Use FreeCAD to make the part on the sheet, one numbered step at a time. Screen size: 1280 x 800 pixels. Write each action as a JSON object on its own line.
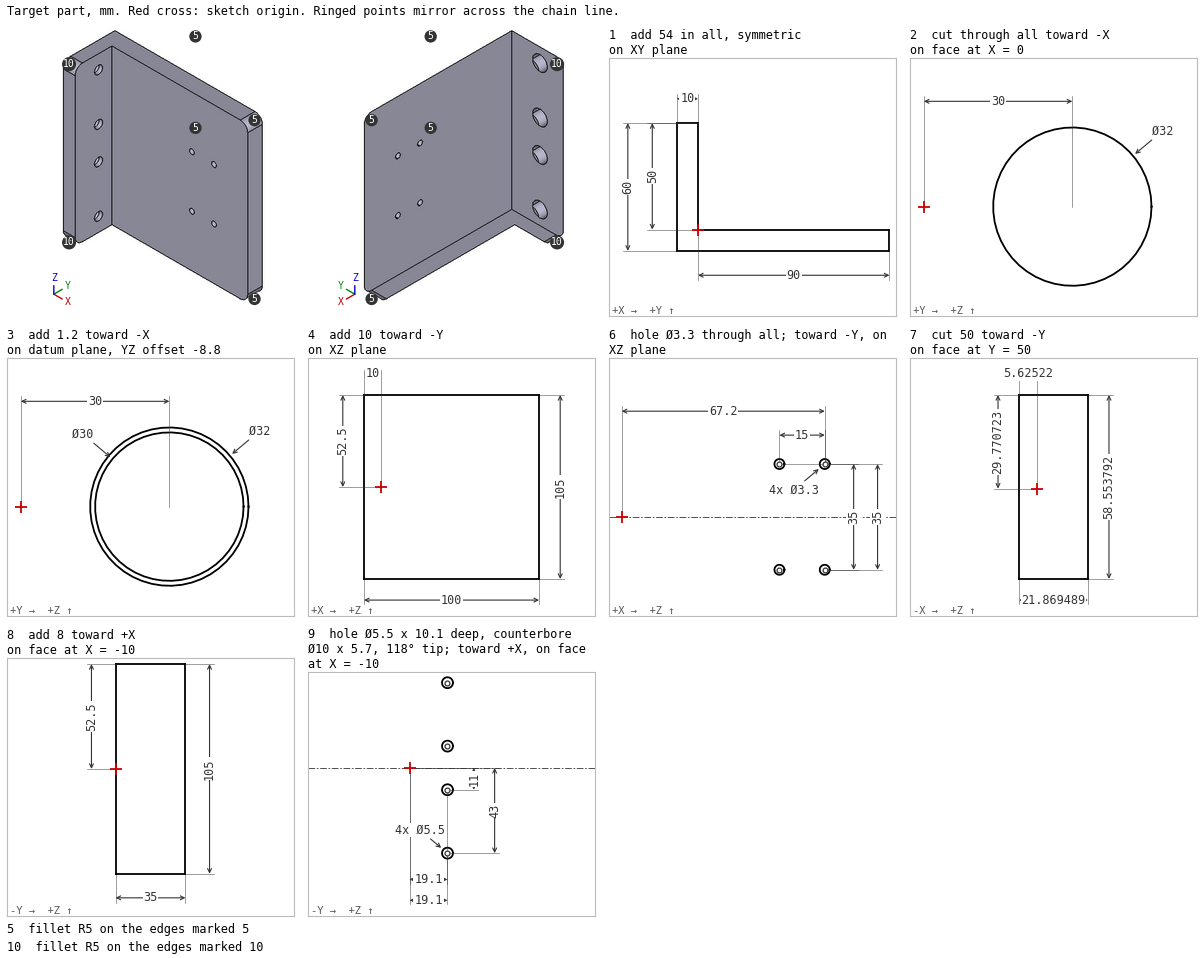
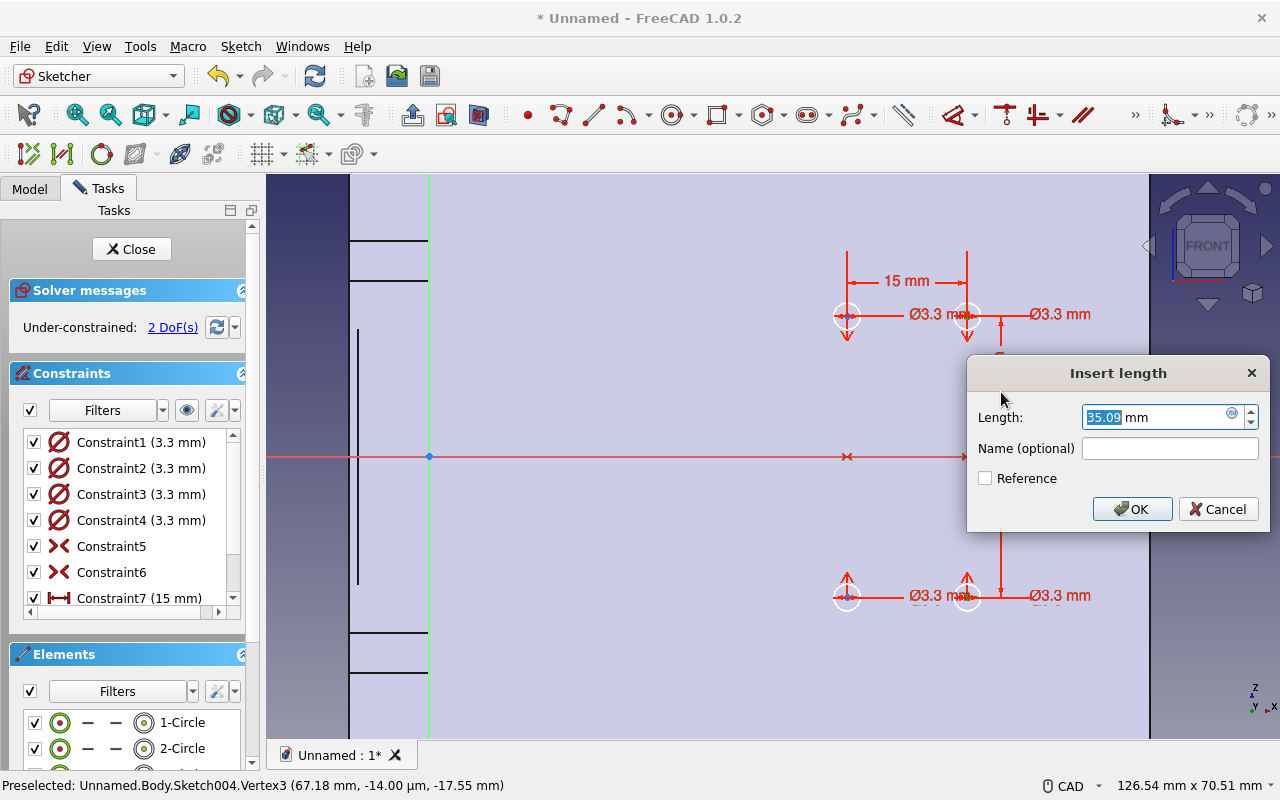
{"action": "type", "text": "35"}
{"action": "key", "text": "Return"}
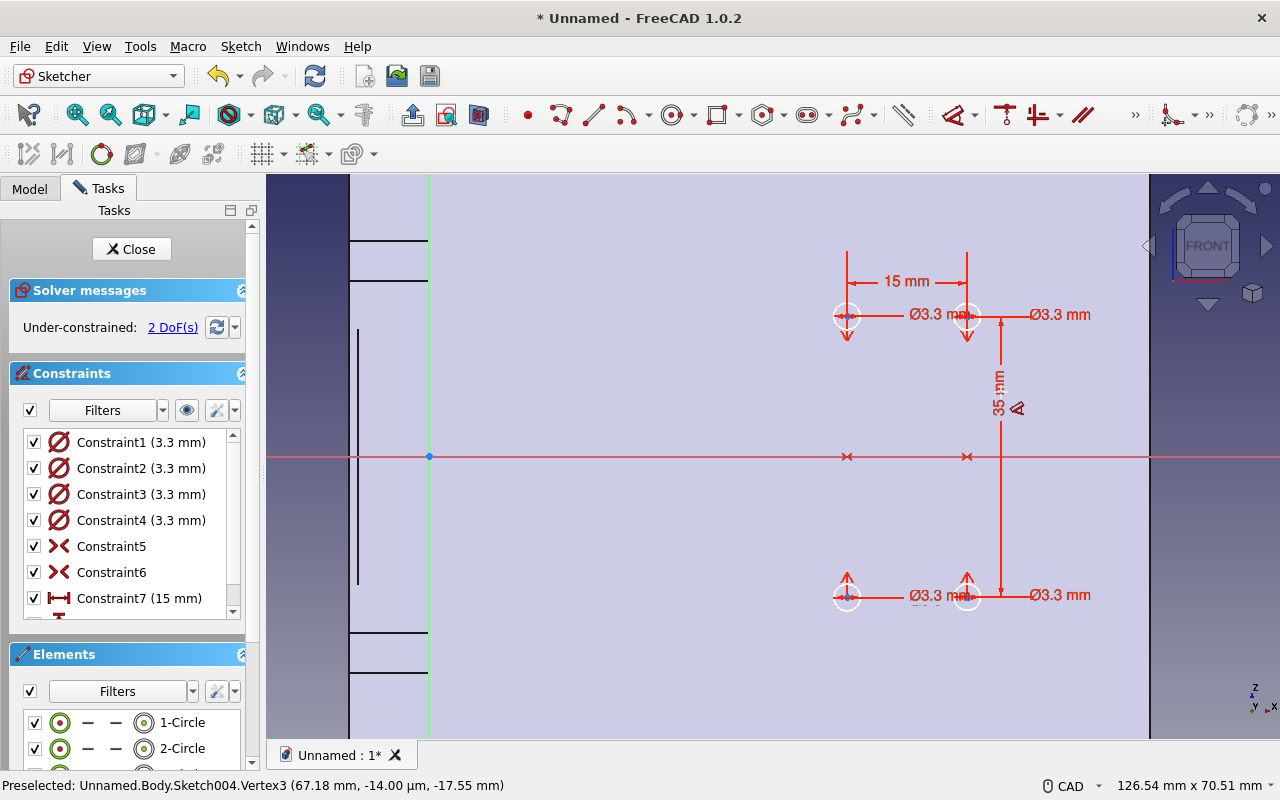
{"action": "left_click", "coordinate": [847, 316]}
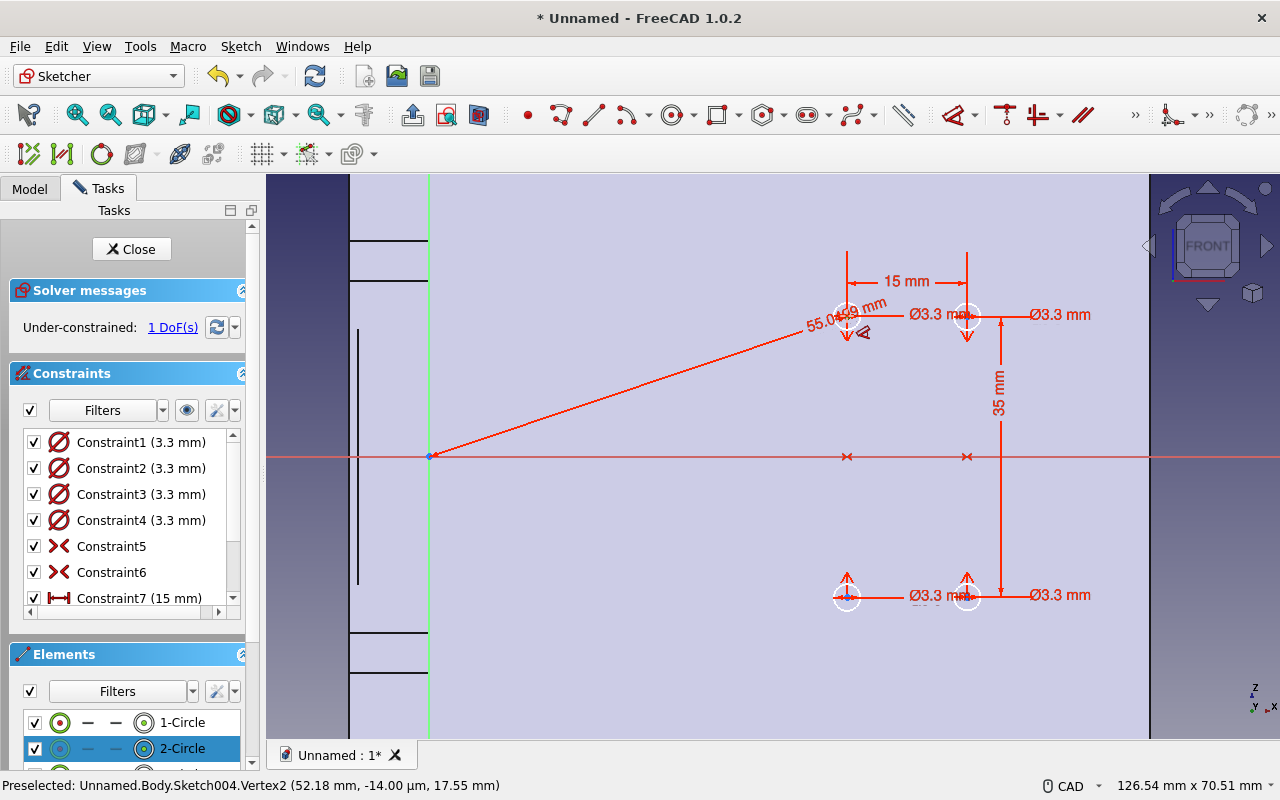
{"action": "left_click", "coordinate": [967, 597]}
{"action": "left_click", "coordinate": [1001, 521]}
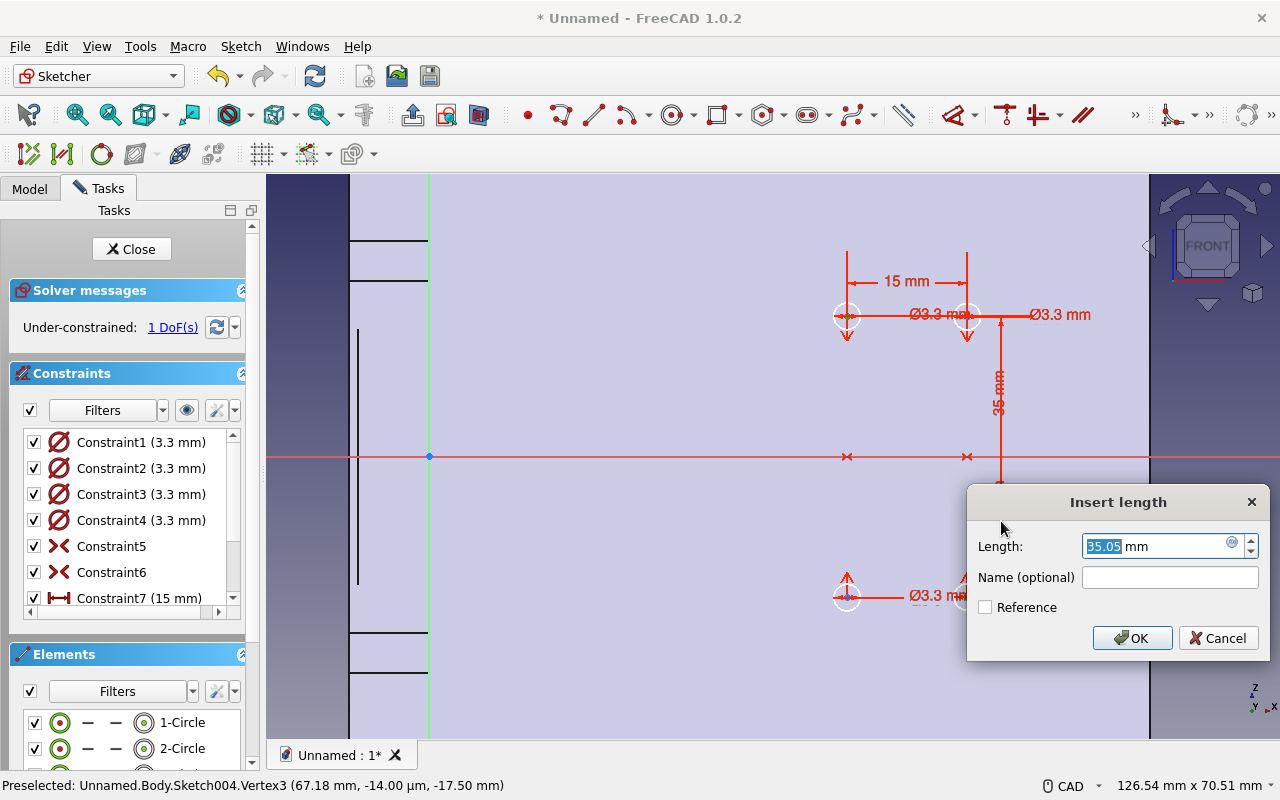
{"action": "type", "text": "35"}
{"action": "key", "text": "Return"}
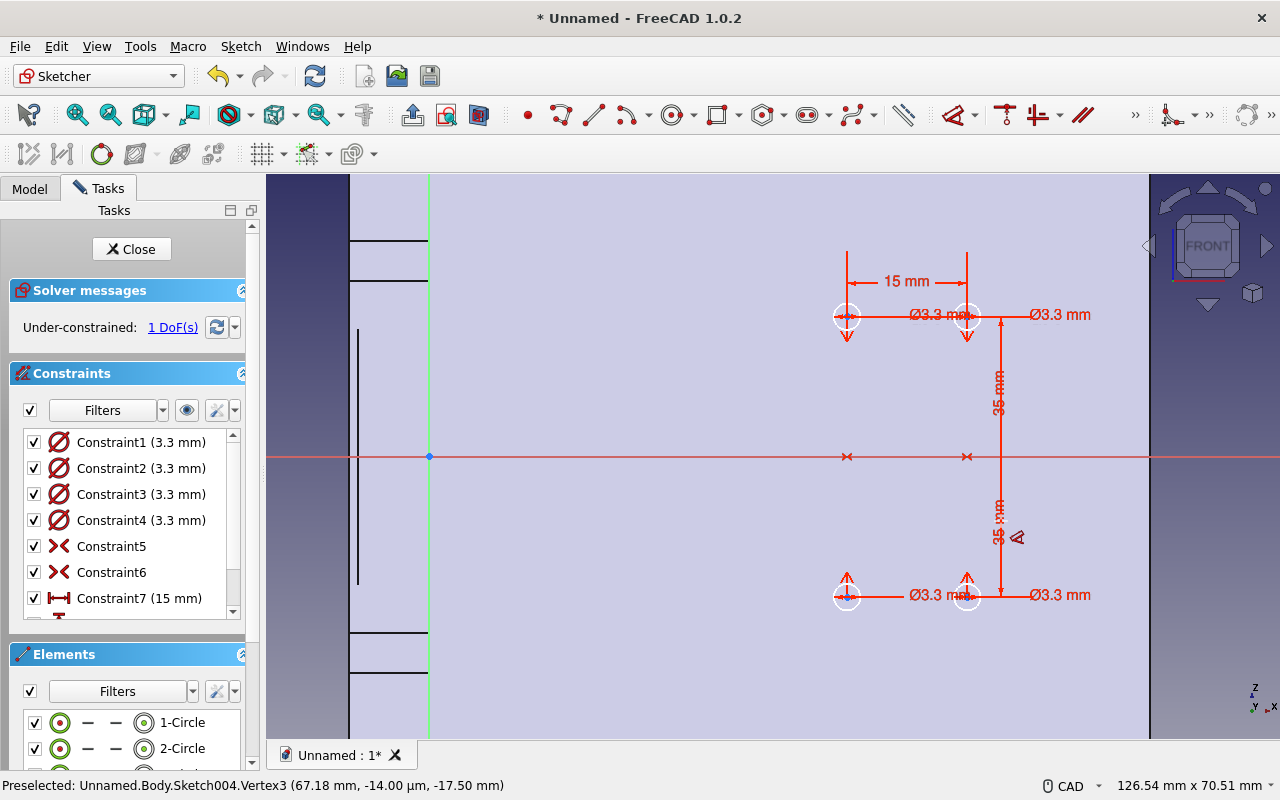
{"action": "left_click", "coordinate": [967, 317]}
{"action": "left_click", "coordinate": [698, 283]}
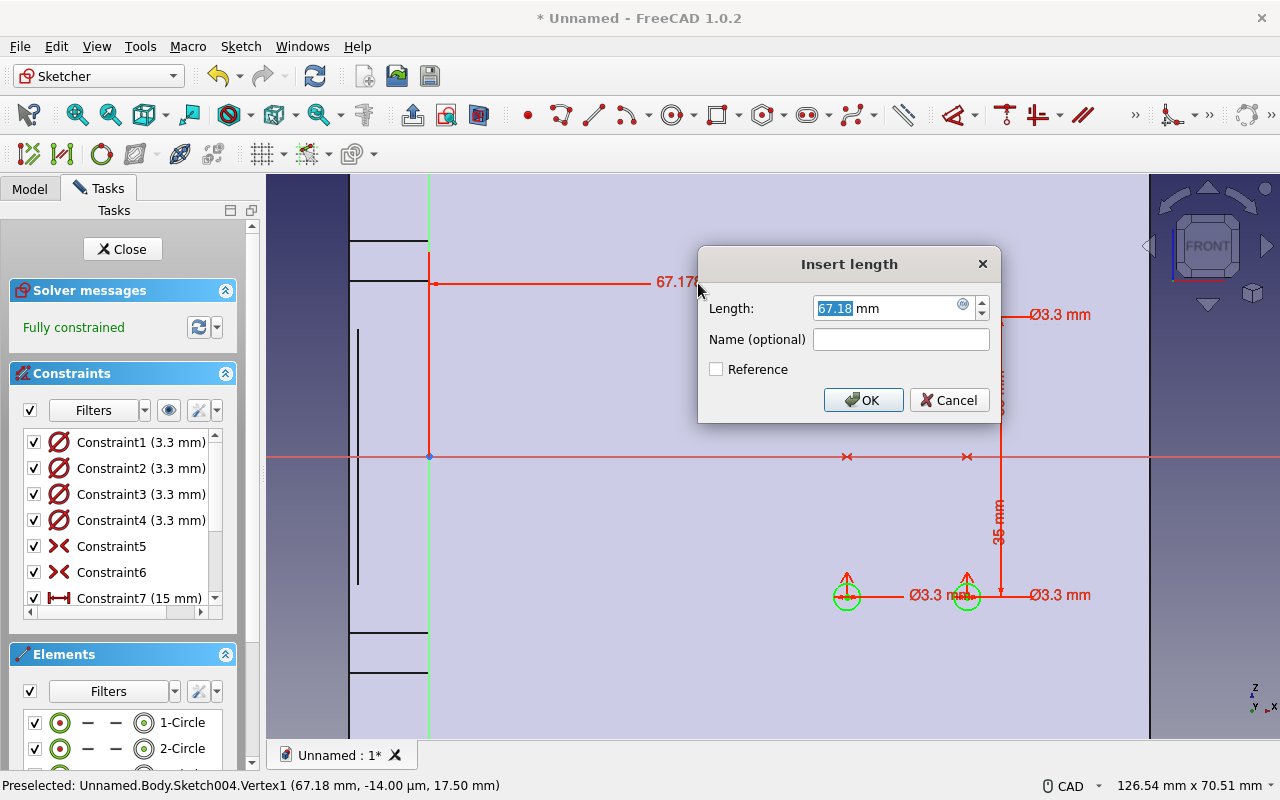
{"action": "type", "text": "67.2"}
{"action": "key", "text": "Return"}
{"action": "key", "text": "Escape"}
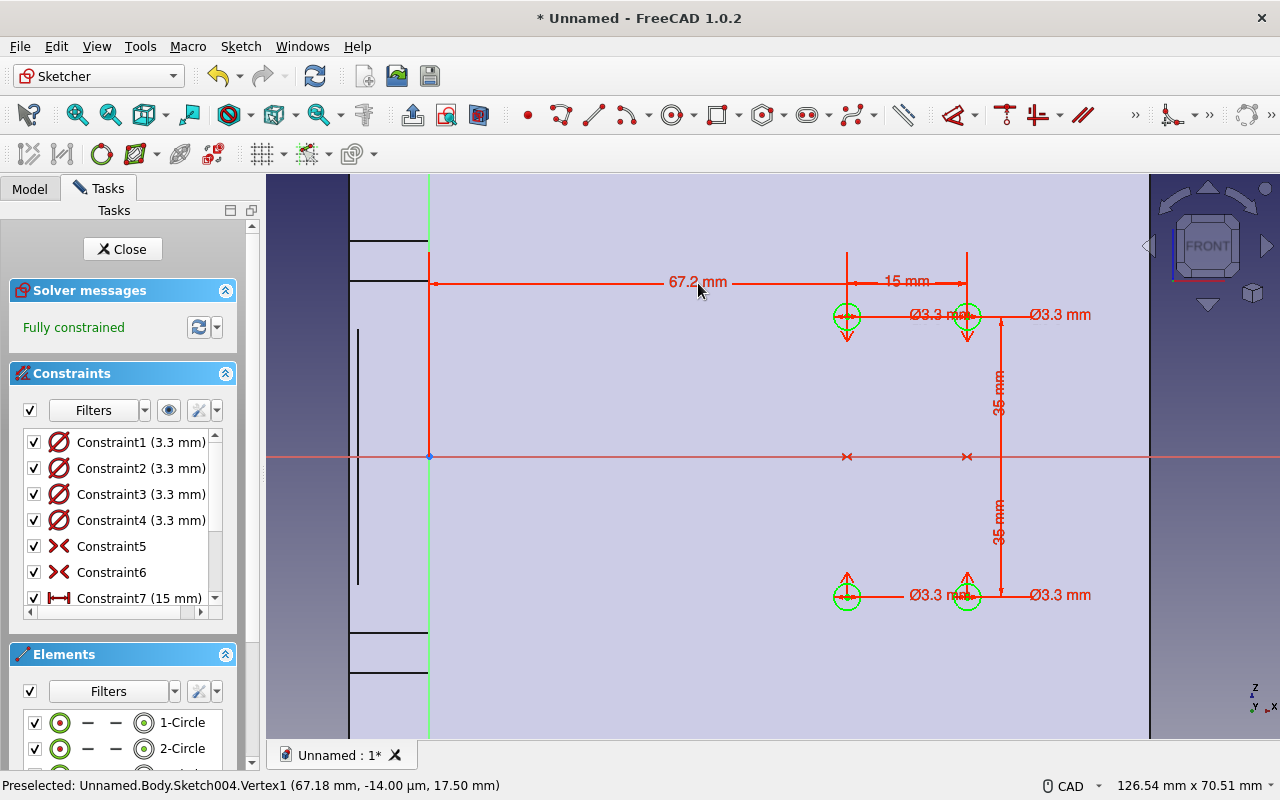
{"action": "left_click", "coordinate": [123, 249]}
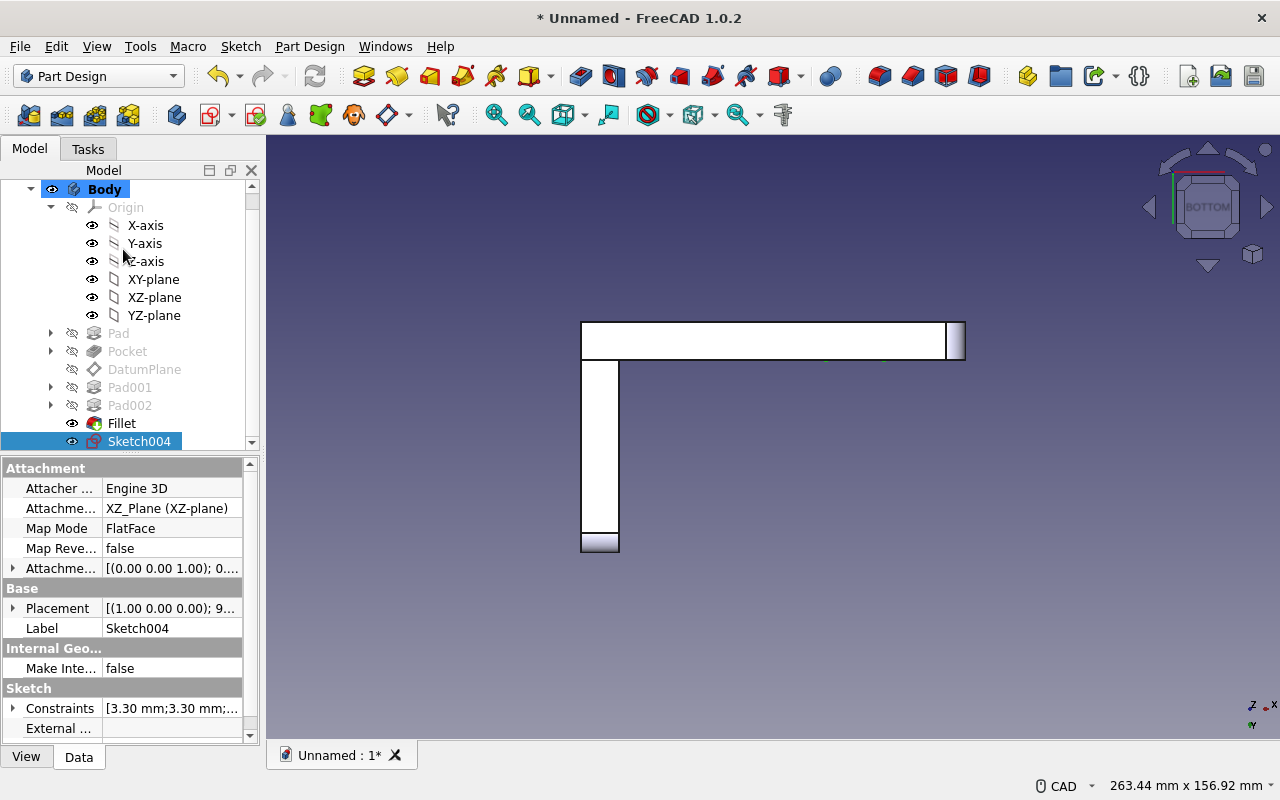
{"action": "left_click", "coordinate": [614, 76]}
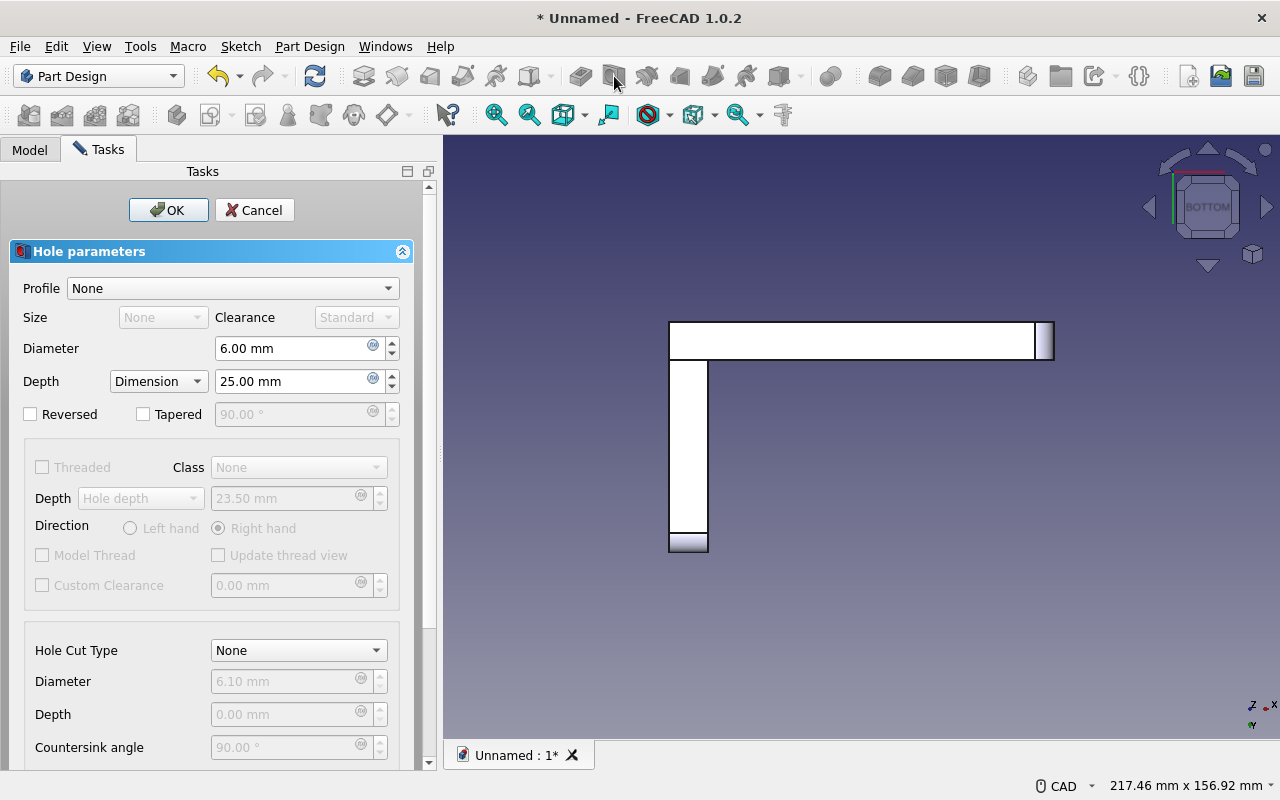
{"action": "triple_click", "coordinate": [300, 348]}